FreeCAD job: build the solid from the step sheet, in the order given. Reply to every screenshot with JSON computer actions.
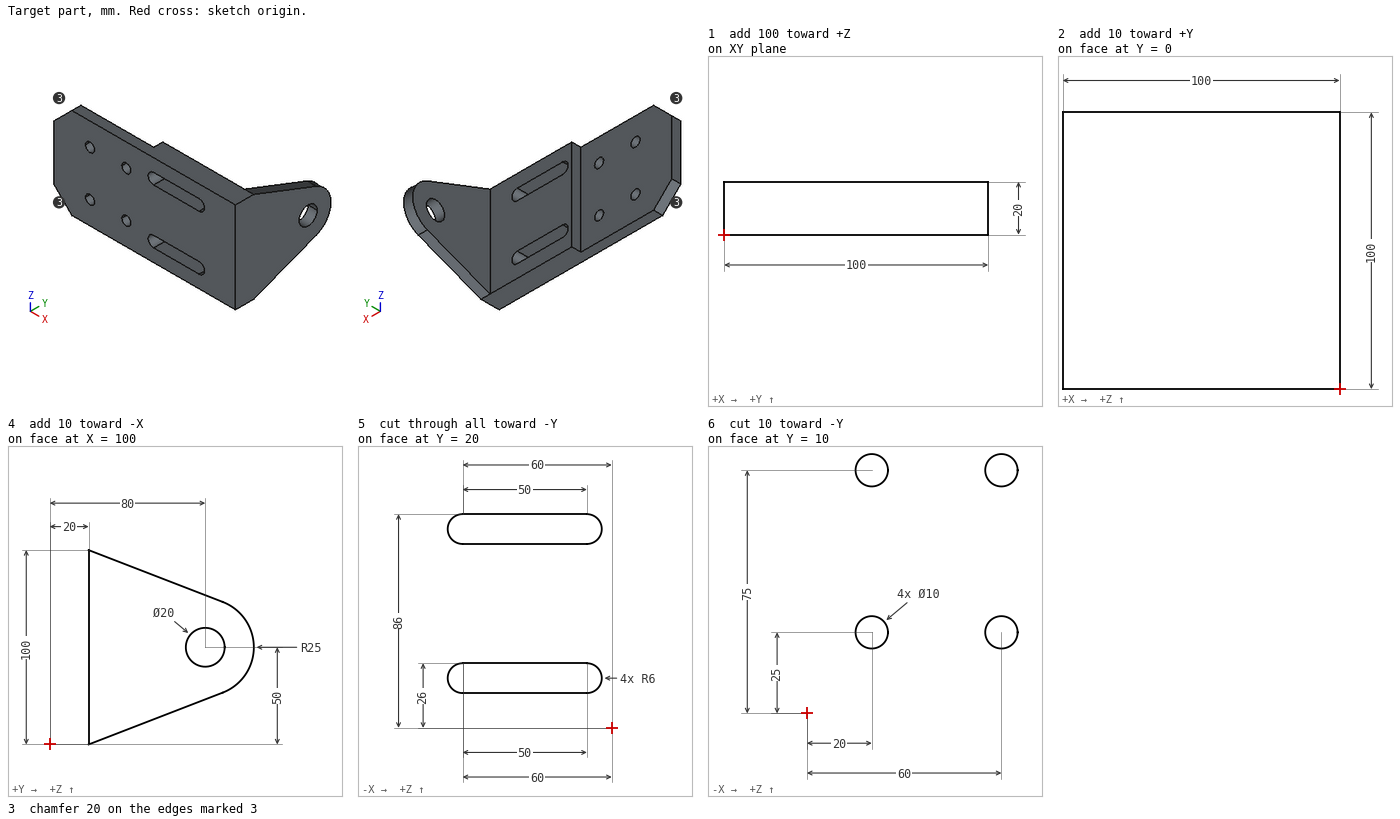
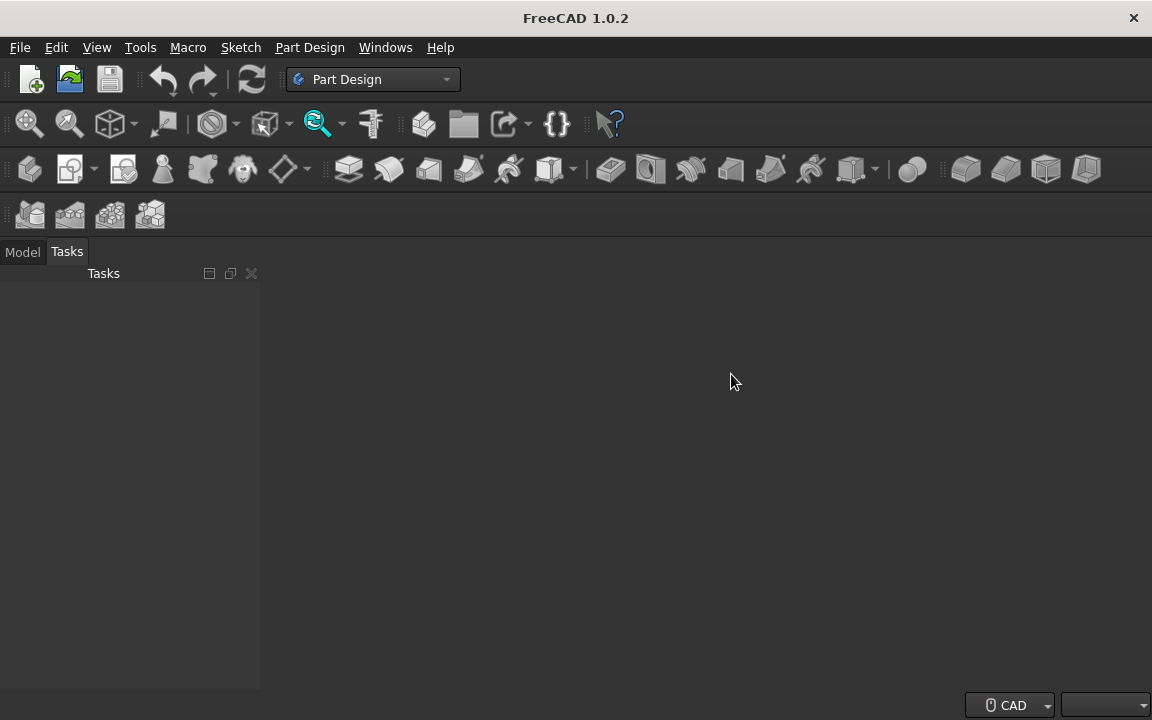
{"action": "left_click", "coordinate": [30, 80]}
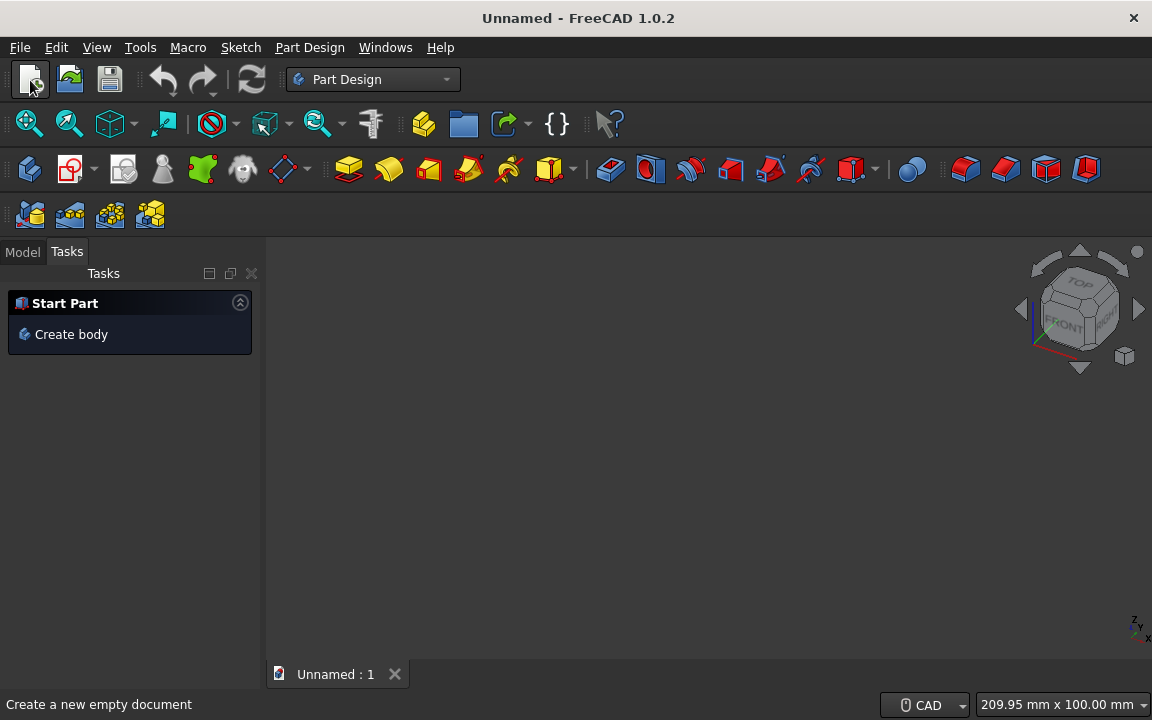
{"action": "left_click", "coordinate": [70, 170]}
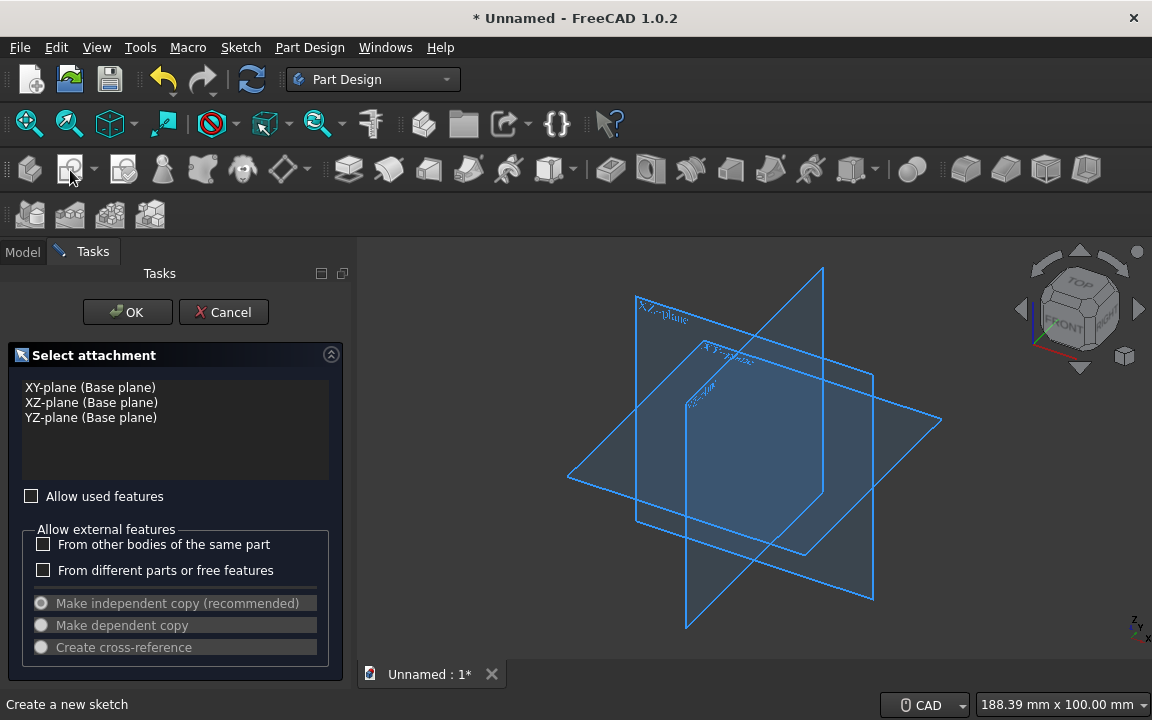
{"action": "left_click", "coordinate": [82, 388]}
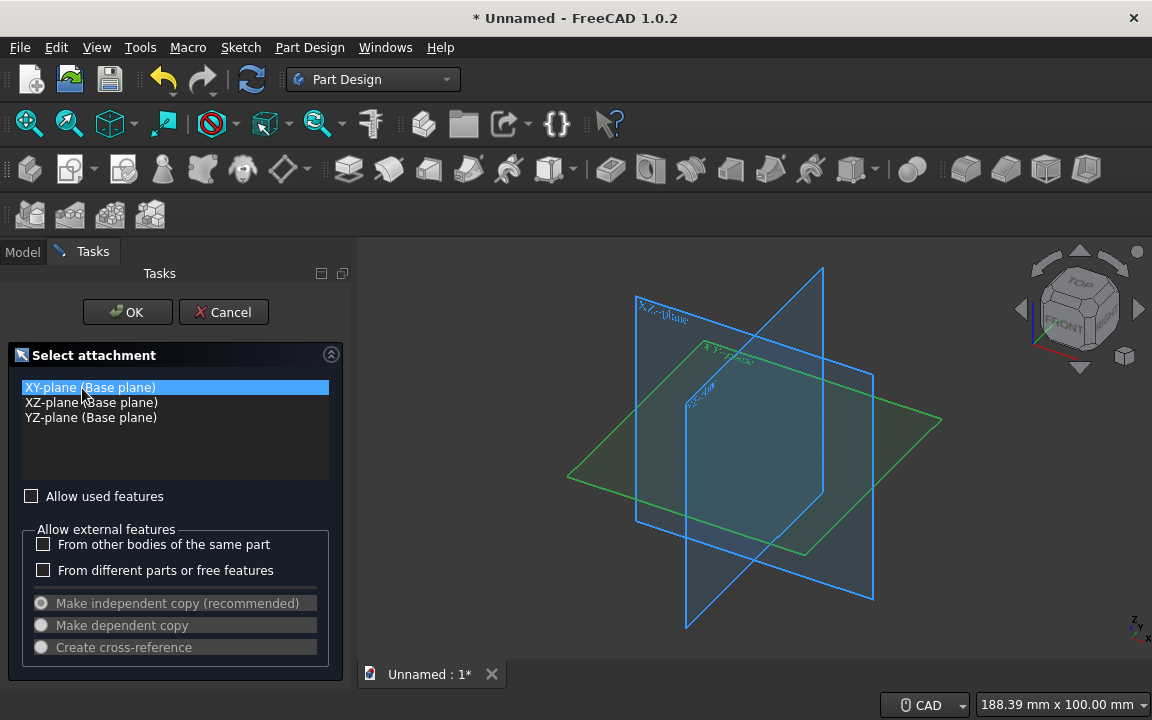
{"action": "left_click", "coordinate": [128, 312]}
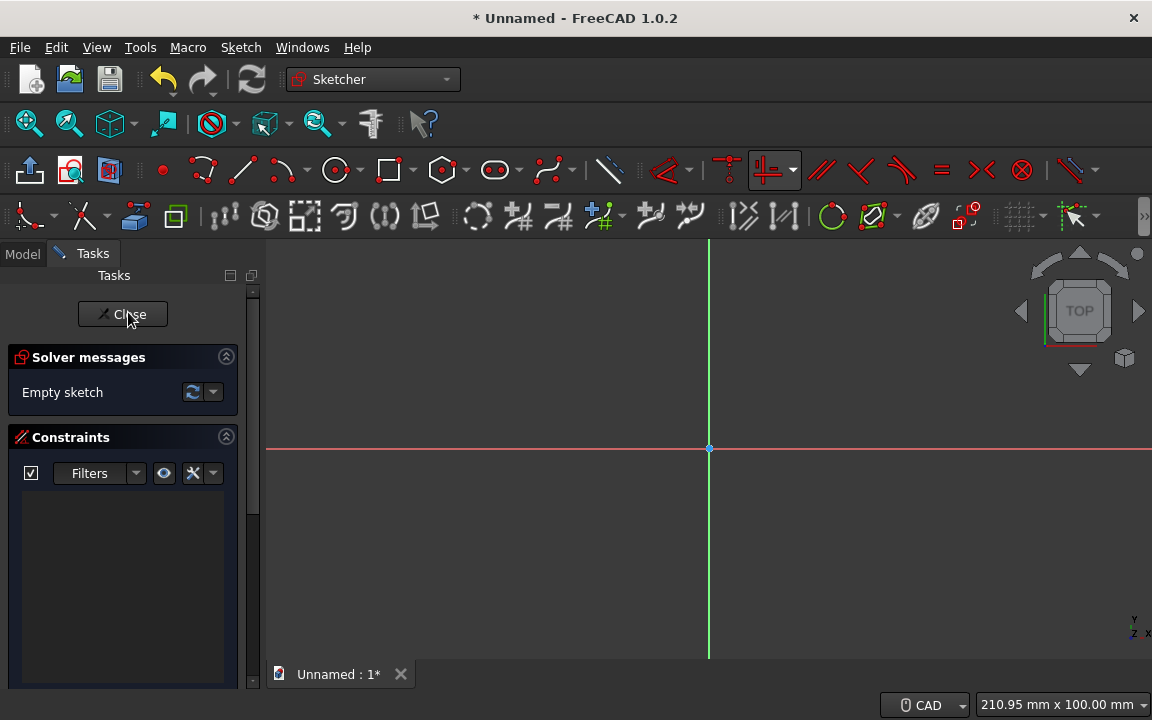
{"action": "scroll", "coordinate": [294, 534], "scroll_direction": "down", "scroll_amount": 2}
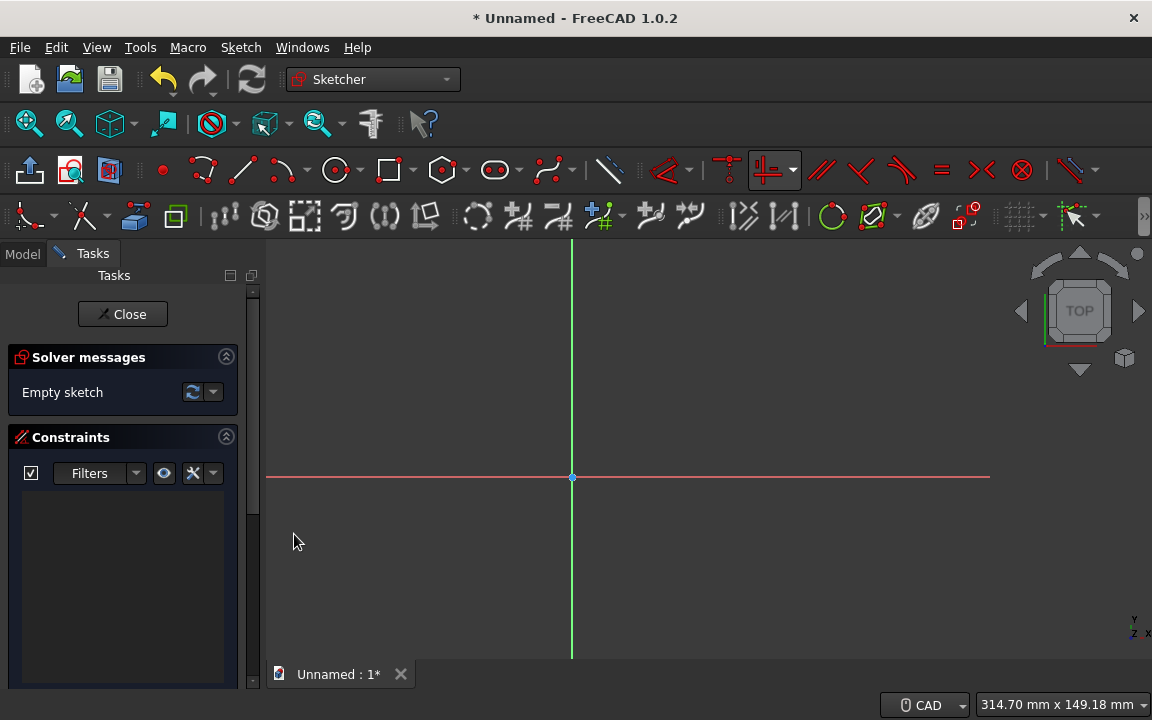
{"action": "scroll", "coordinate": [801, 449], "scroll_direction": "up", "scroll_amount": 3}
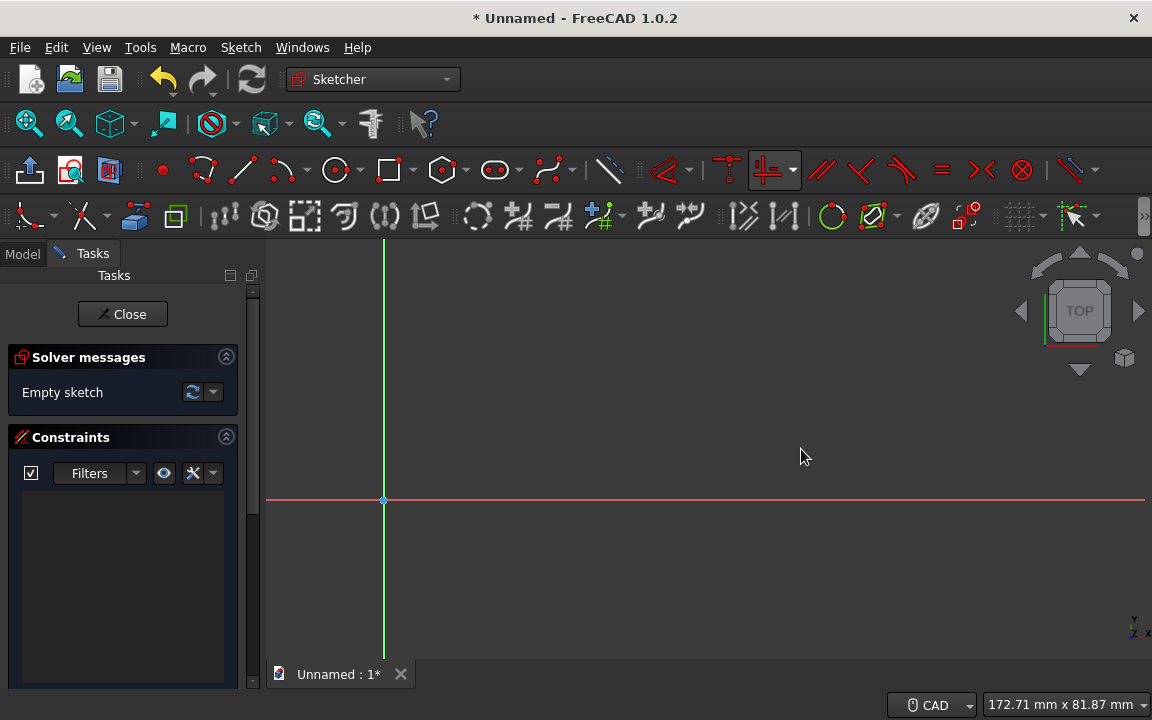
{"action": "left_click", "coordinate": [390, 170]}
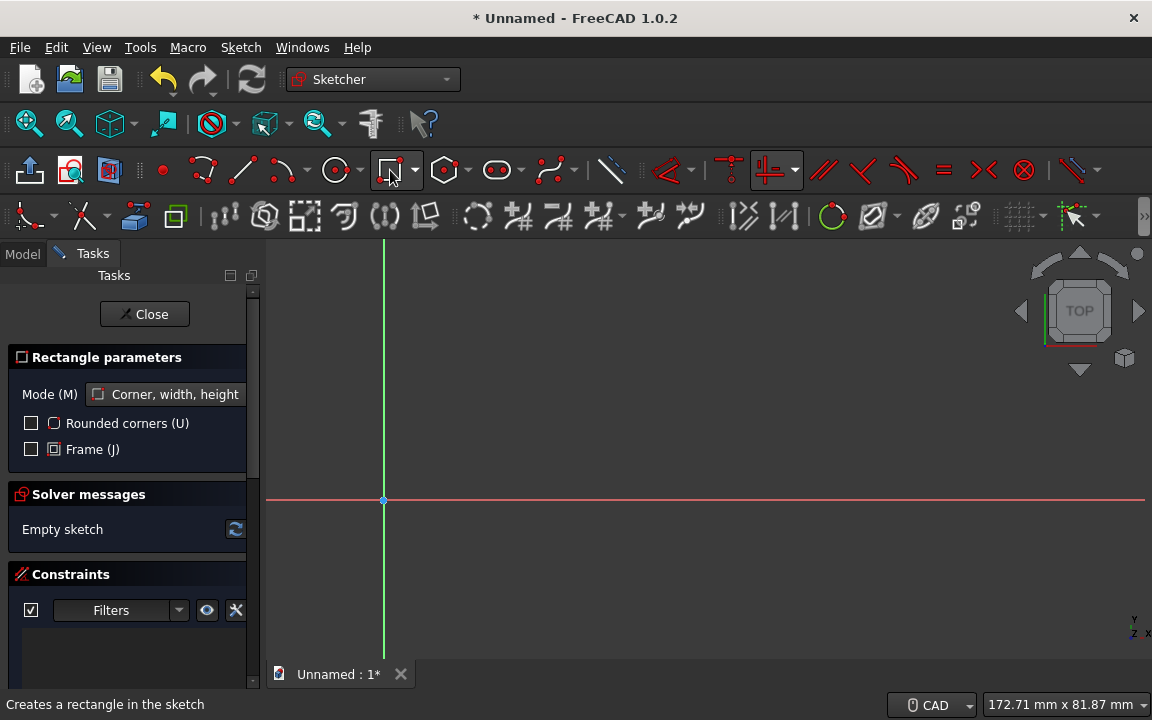
{"action": "left_click", "coordinate": [384, 500]}
{"action": "left_click", "coordinate": [897, 397]}
{"action": "key", "text": "Escape"}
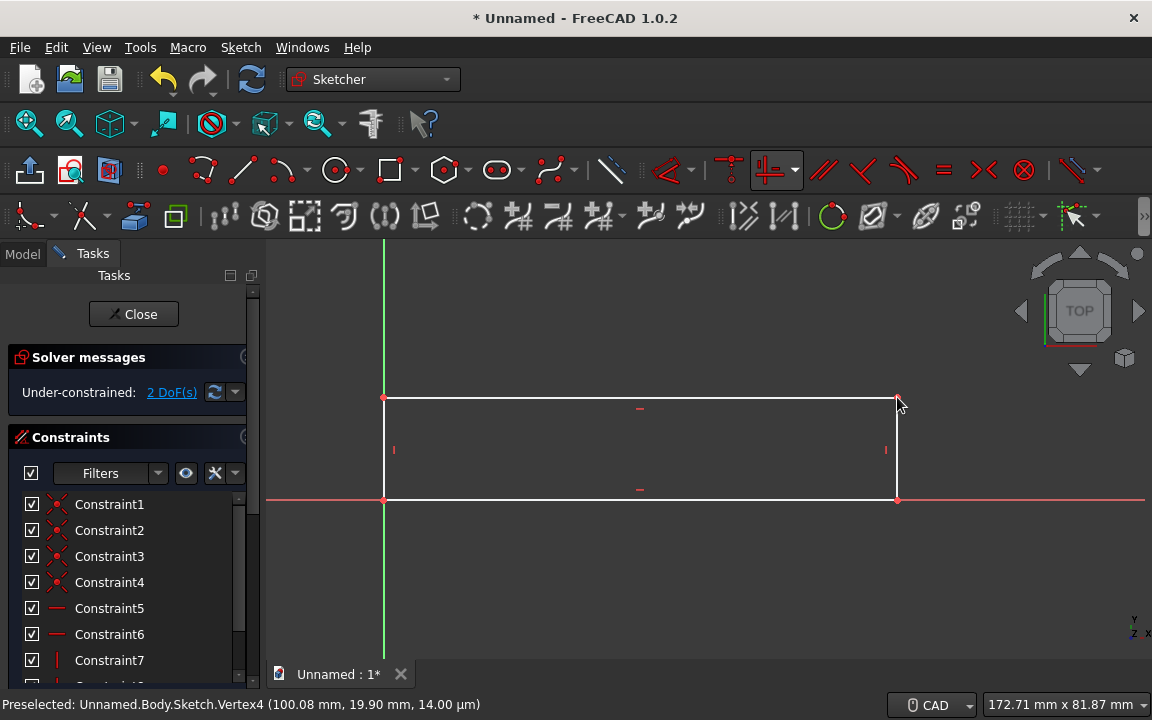
{"action": "left_click", "coordinate": [666, 170]}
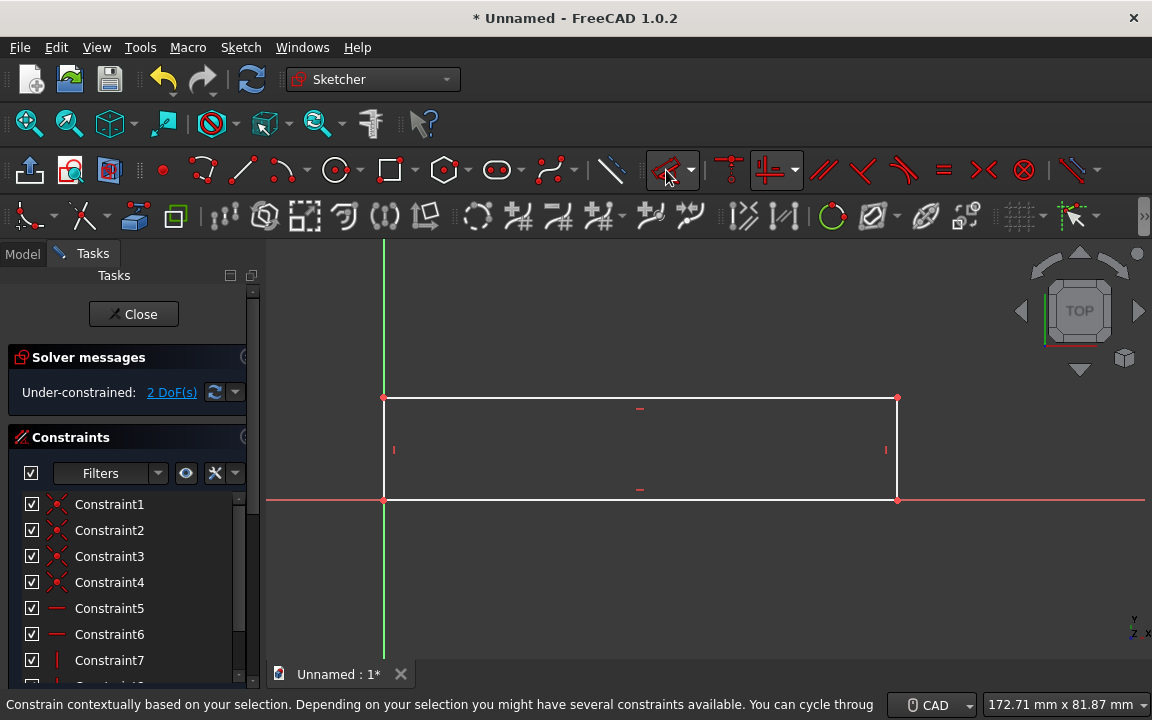
{"action": "left_click", "coordinate": [897, 469]}
{"action": "left_click", "coordinate": [931, 449]}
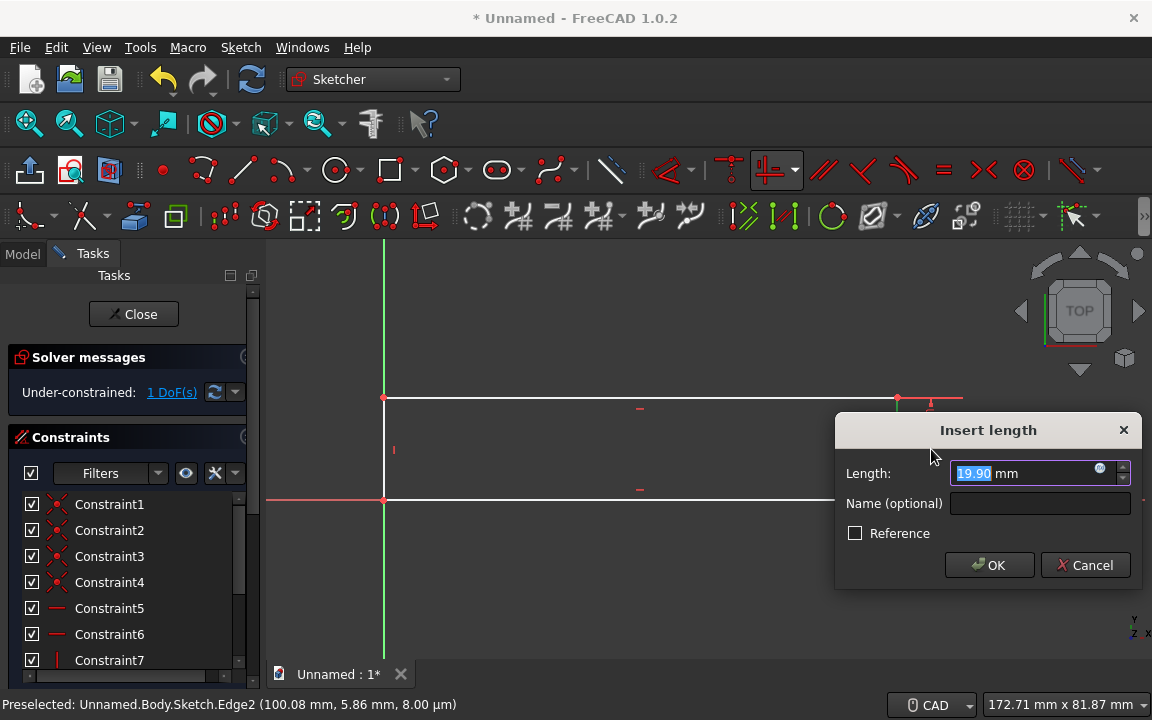
{"action": "type", "text": "20"}
{"action": "key", "text": "Return"}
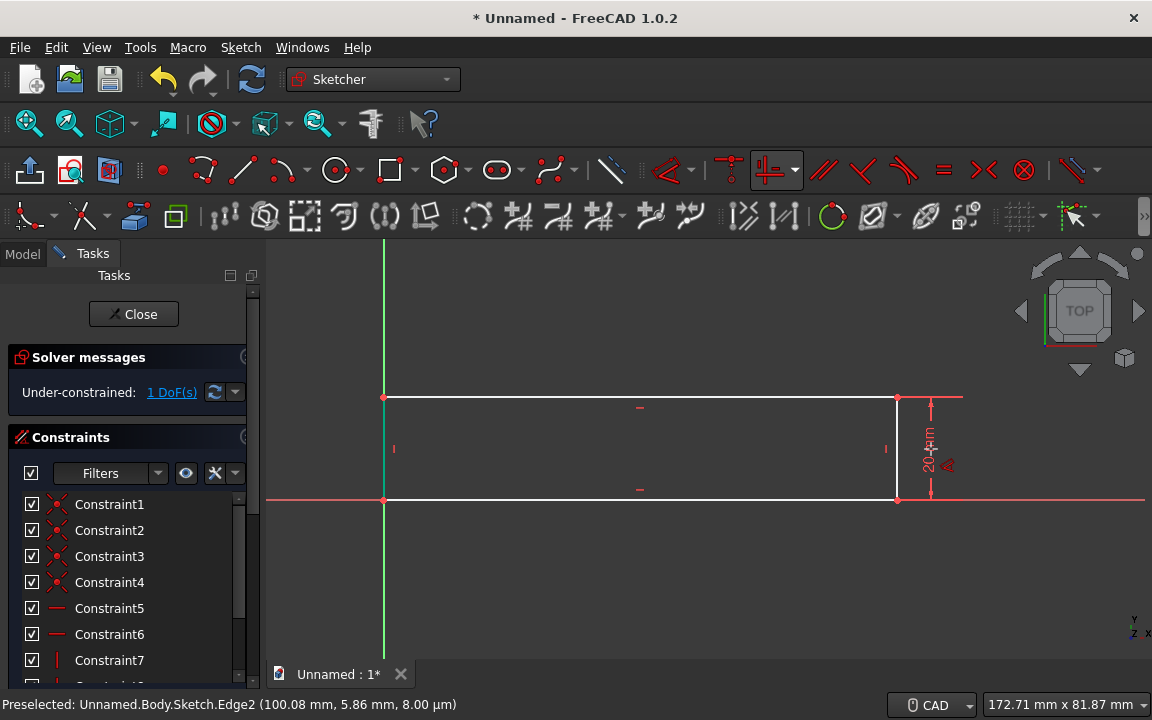
{"action": "left_click", "coordinate": [538, 500]}
{"action": "left_click", "coordinate": [640, 534]}